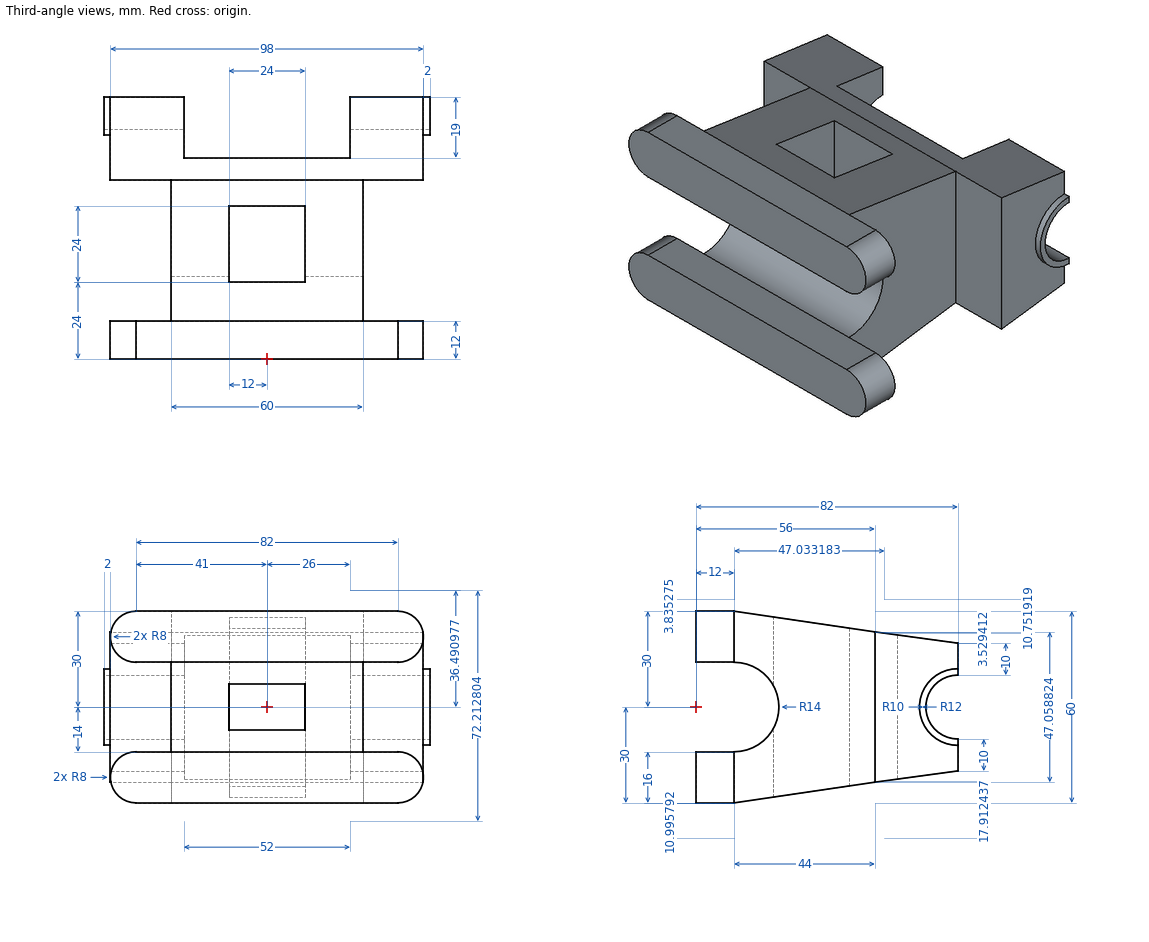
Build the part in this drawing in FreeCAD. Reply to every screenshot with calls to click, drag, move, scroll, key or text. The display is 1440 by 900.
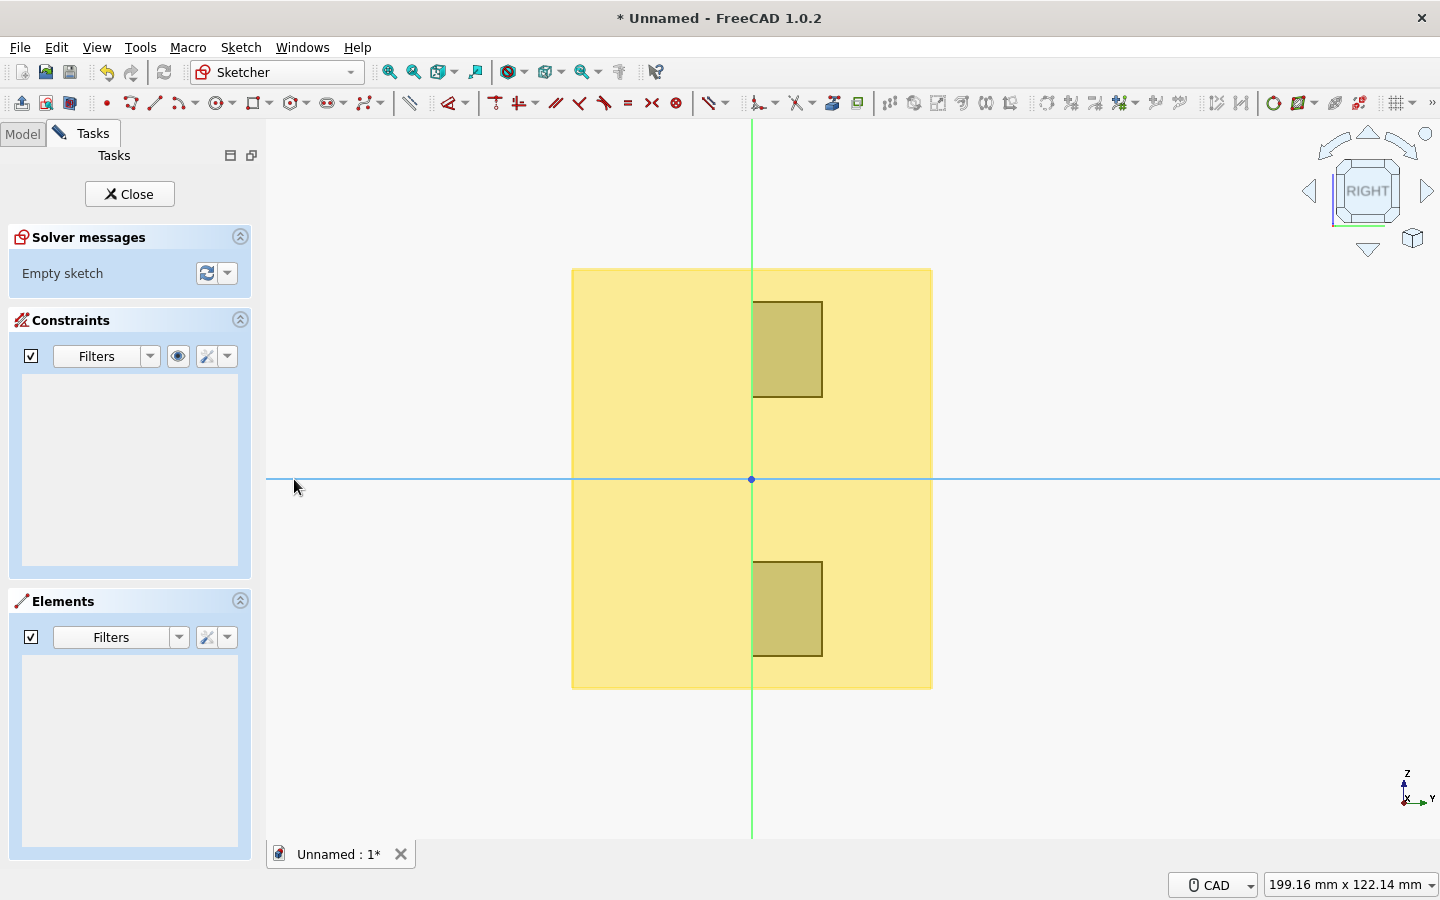
click(132, 104)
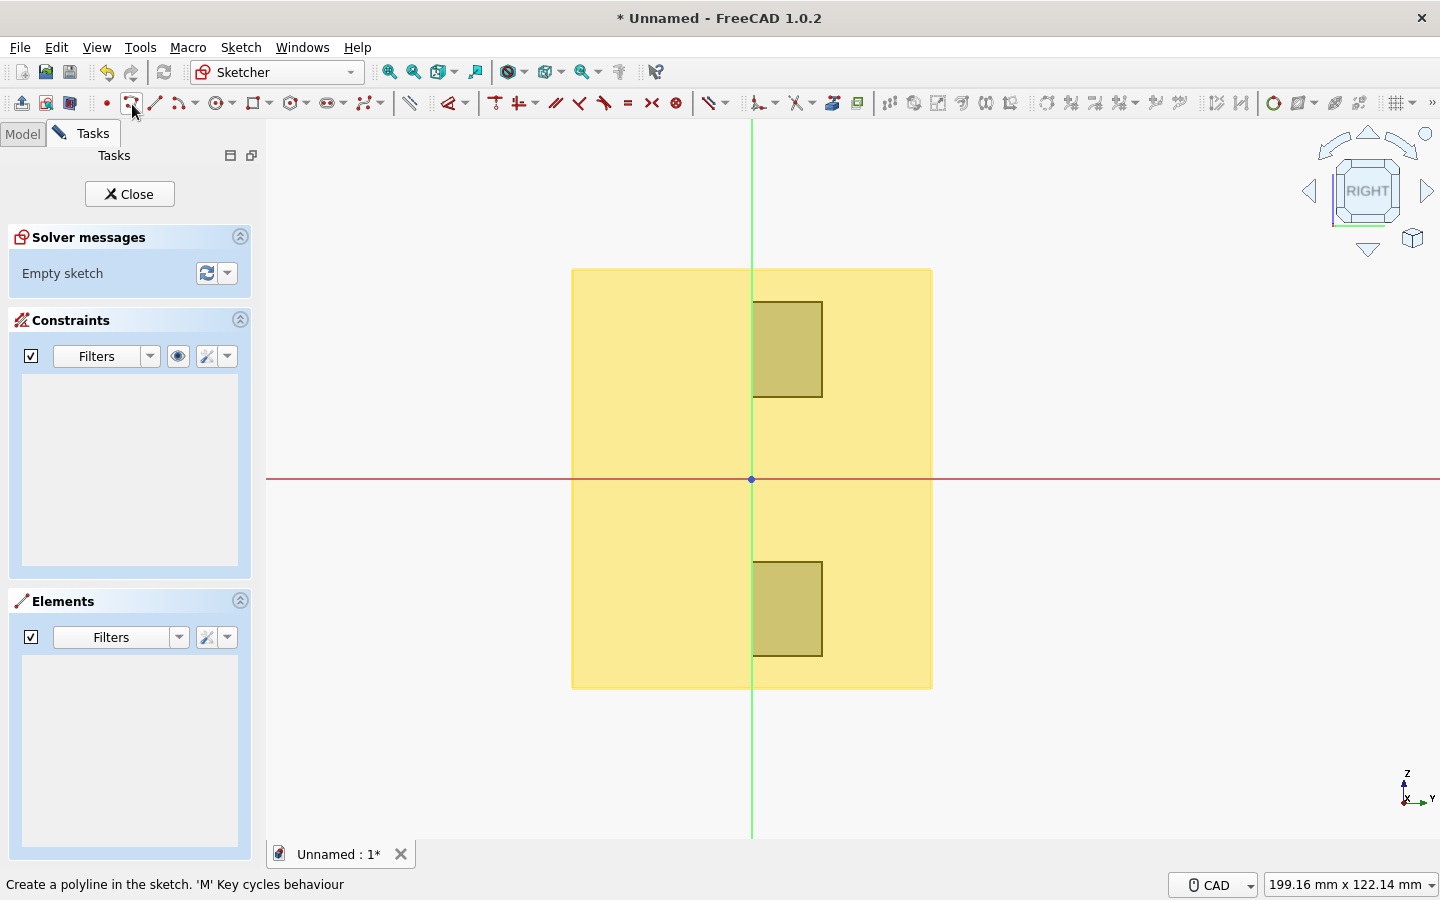
click(822, 562)
click(822, 656)
click(1082, 656)
click(1082, 302)
click(822, 302)
click(822, 397)
right_click(822, 397)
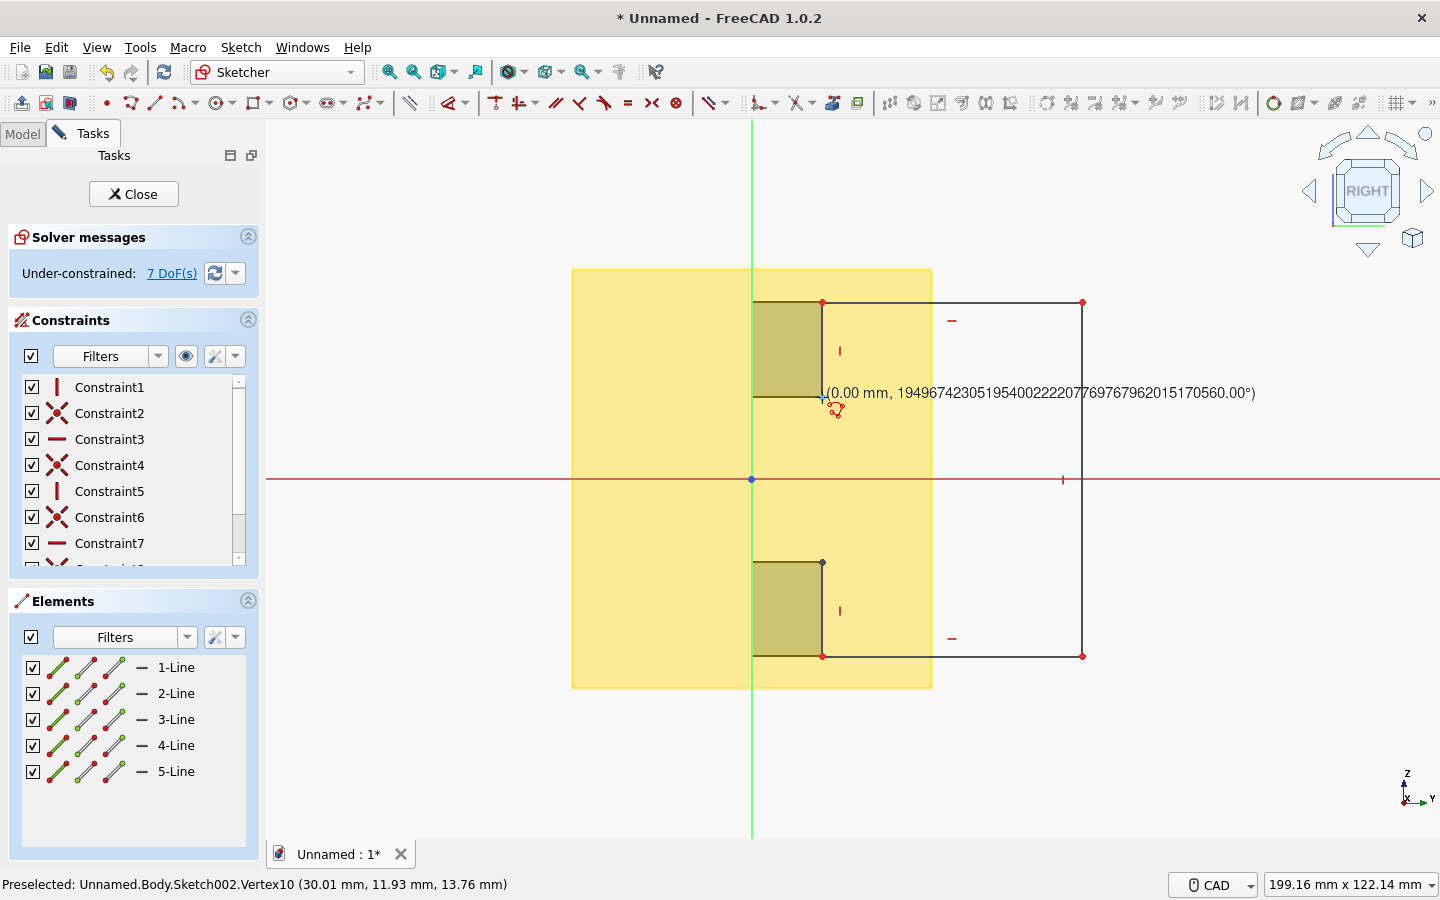
click(198, 104)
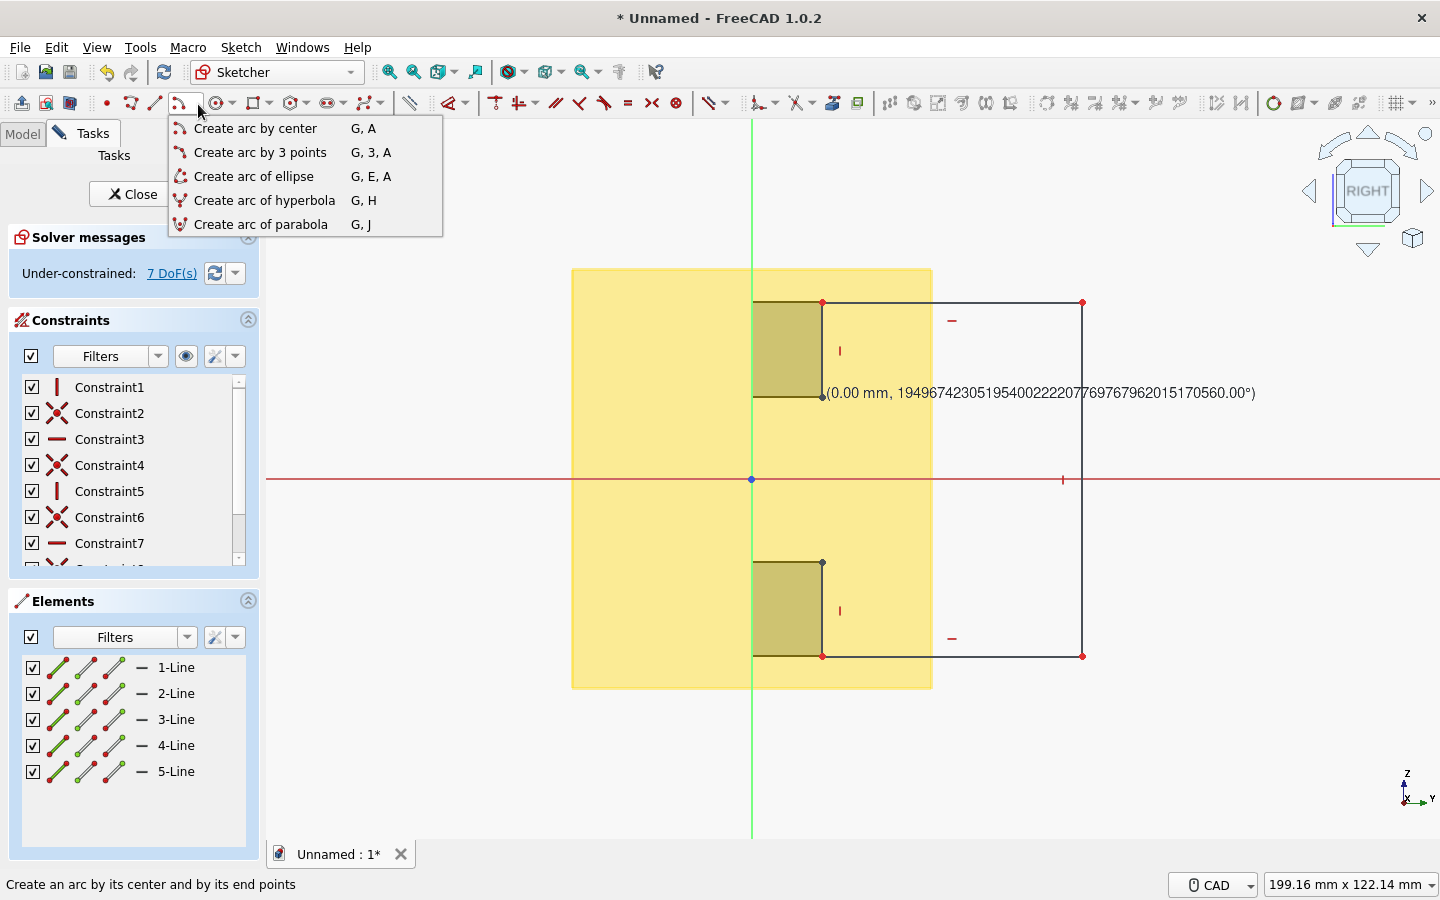
click(306, 152)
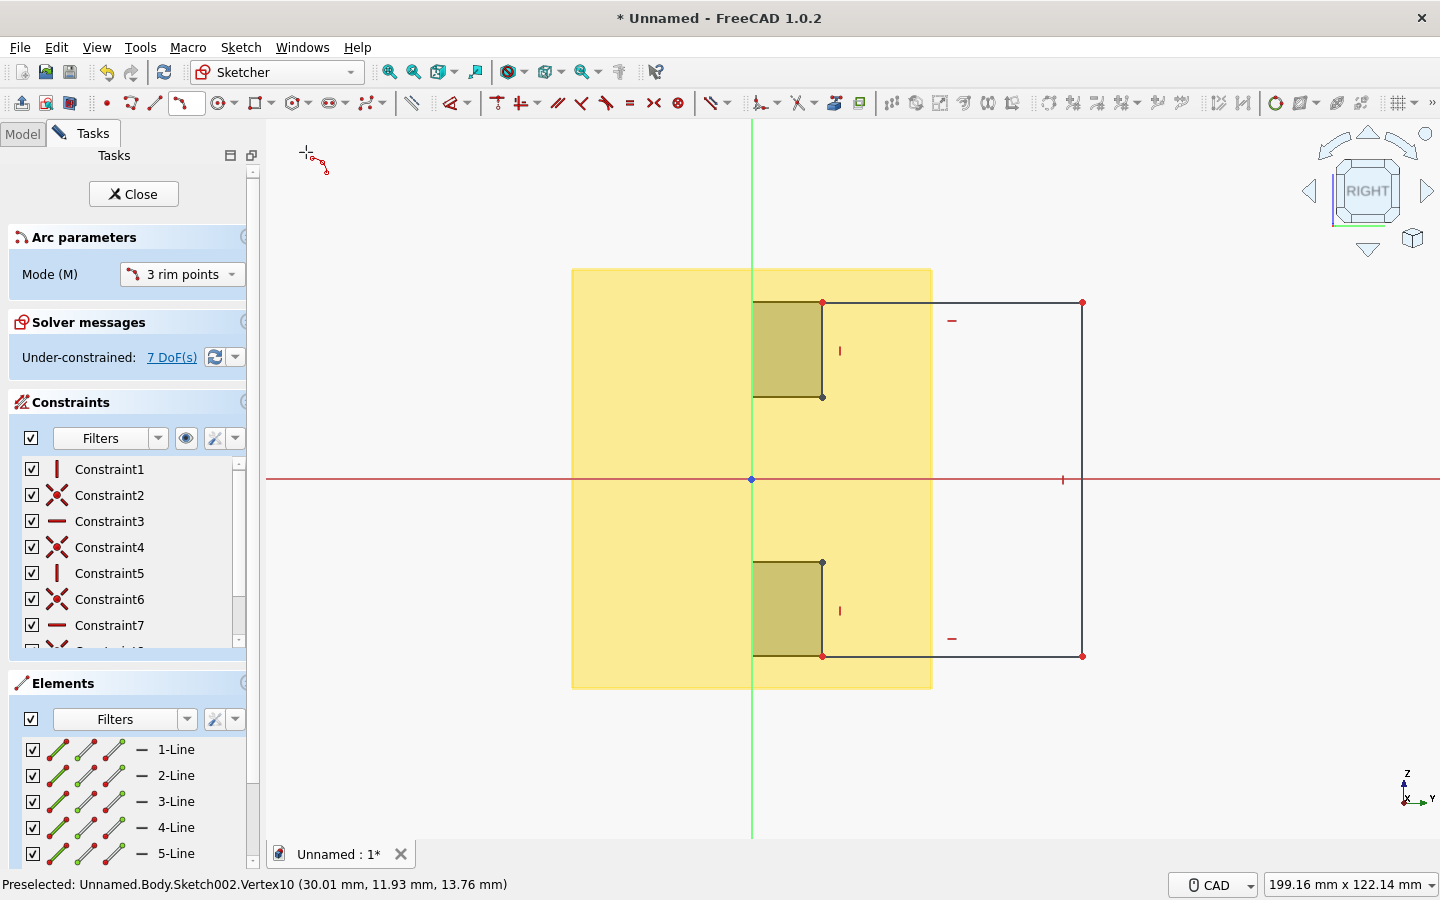
click(822, 398)
click(822, 563)
click(901, 505)
key(Escape)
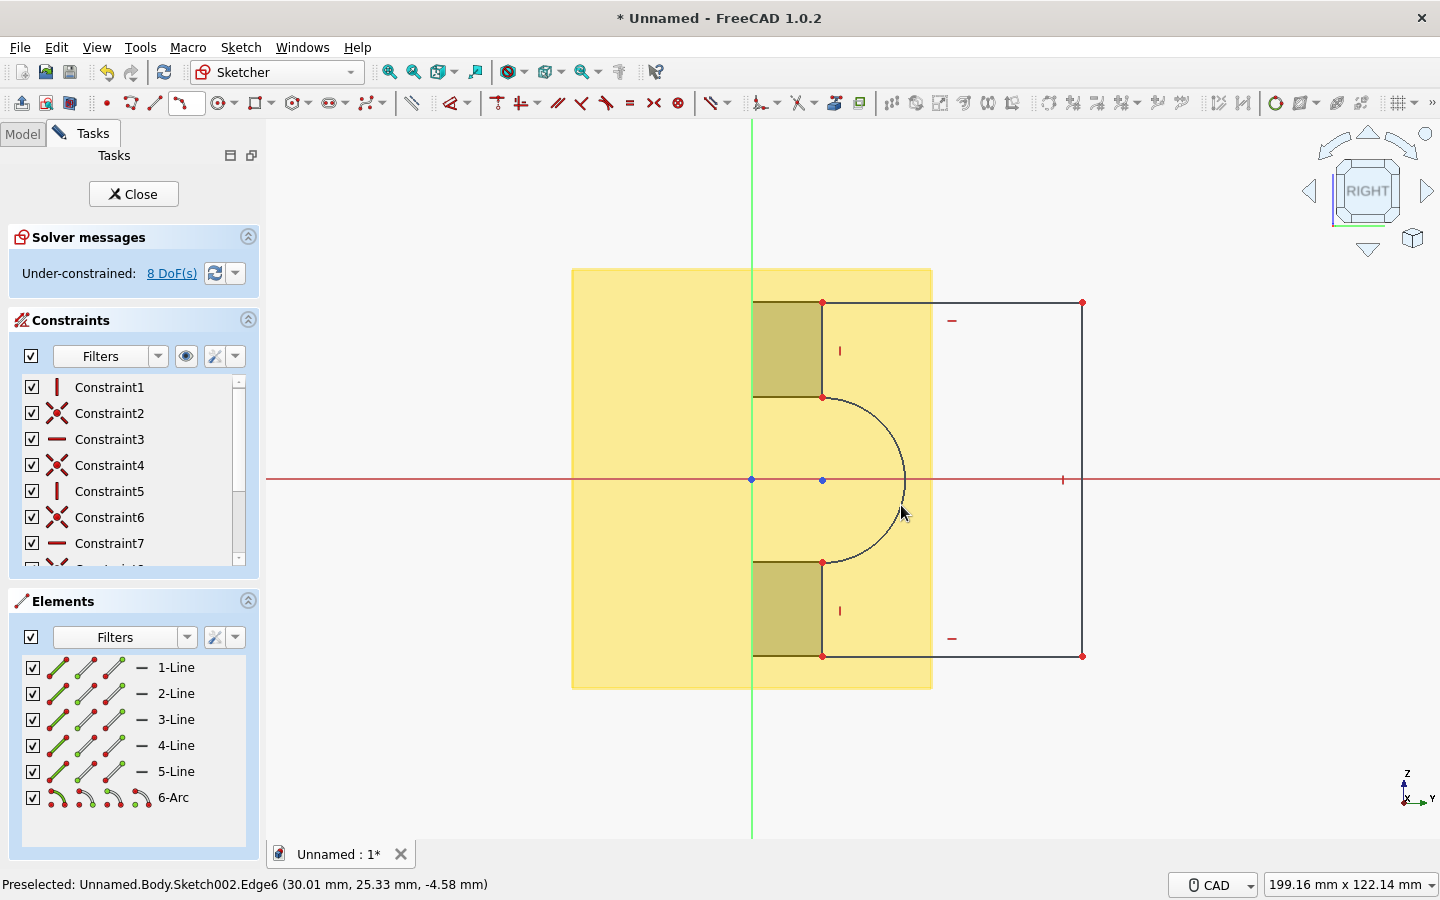
click(823, 480)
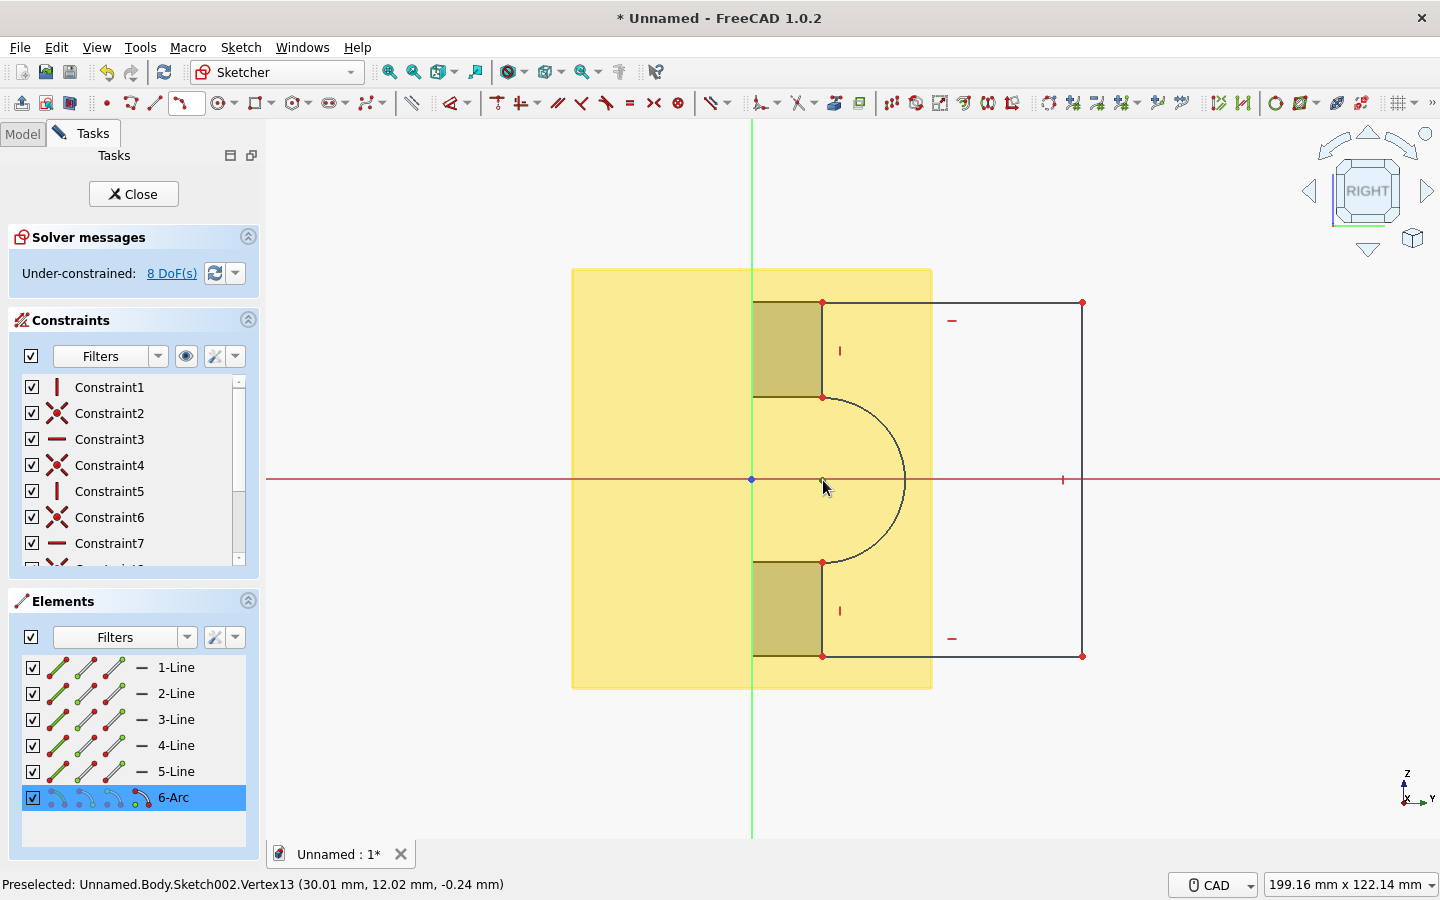
click(364, 479)